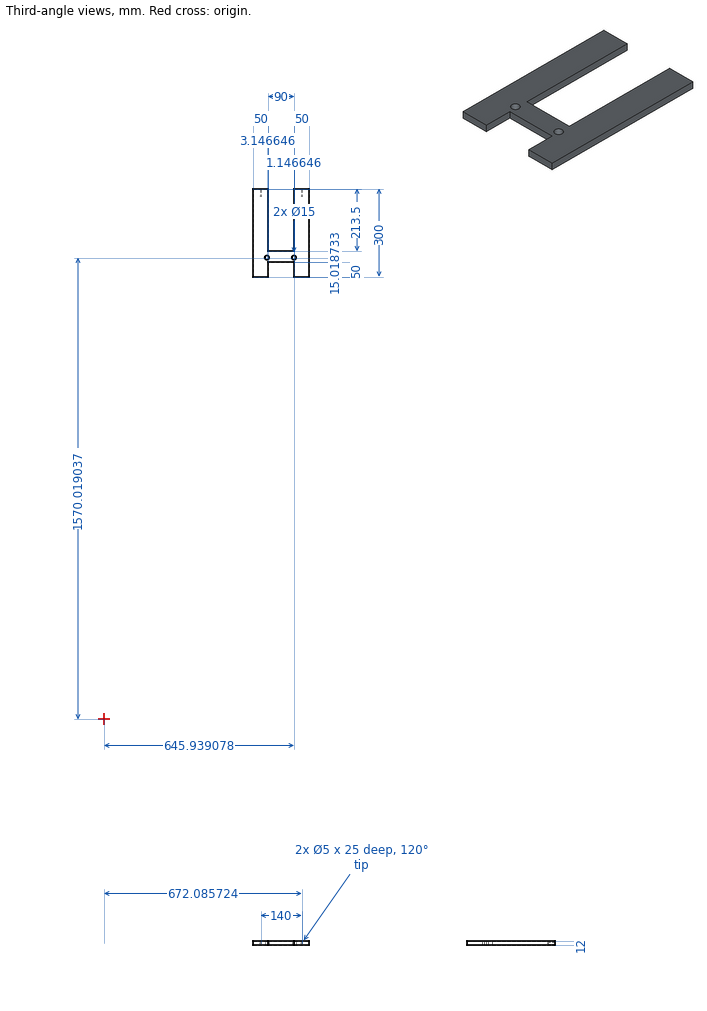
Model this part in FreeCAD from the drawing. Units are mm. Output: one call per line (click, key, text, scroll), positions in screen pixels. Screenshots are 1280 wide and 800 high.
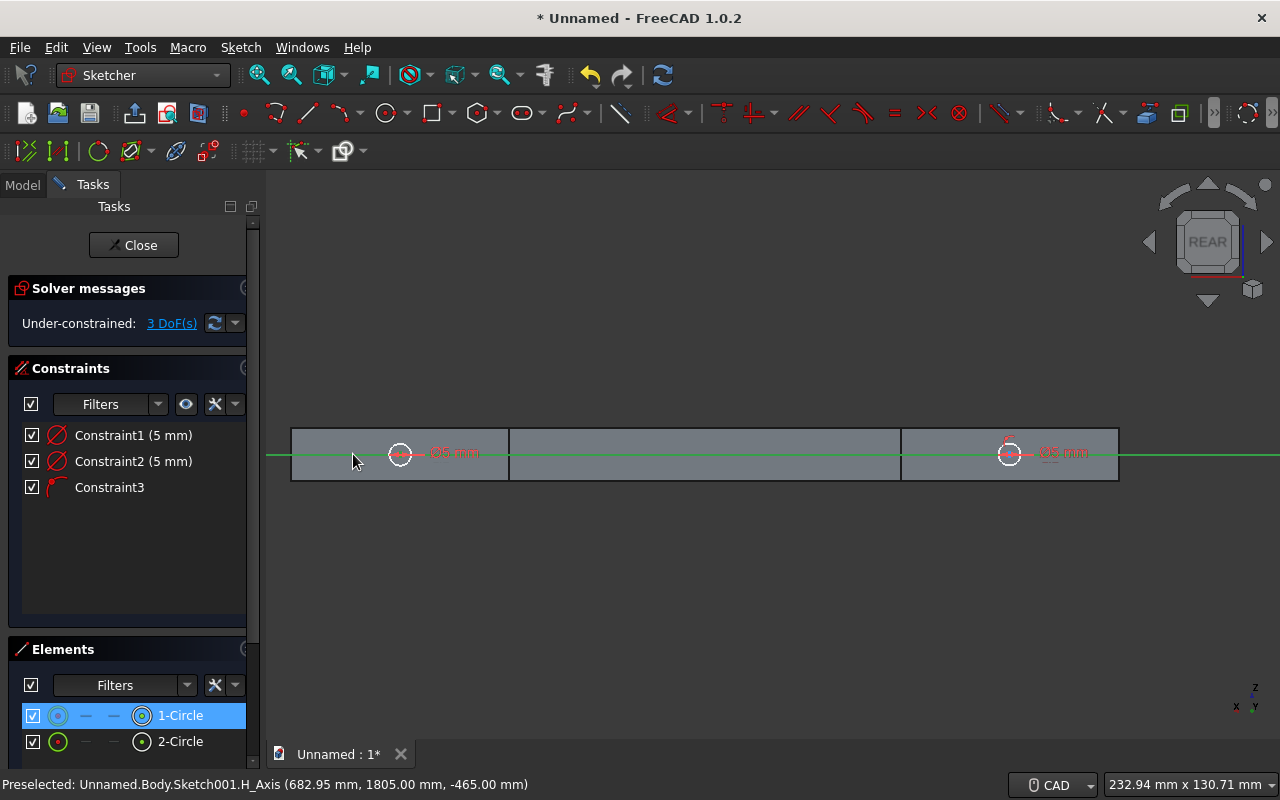
click(722, 114)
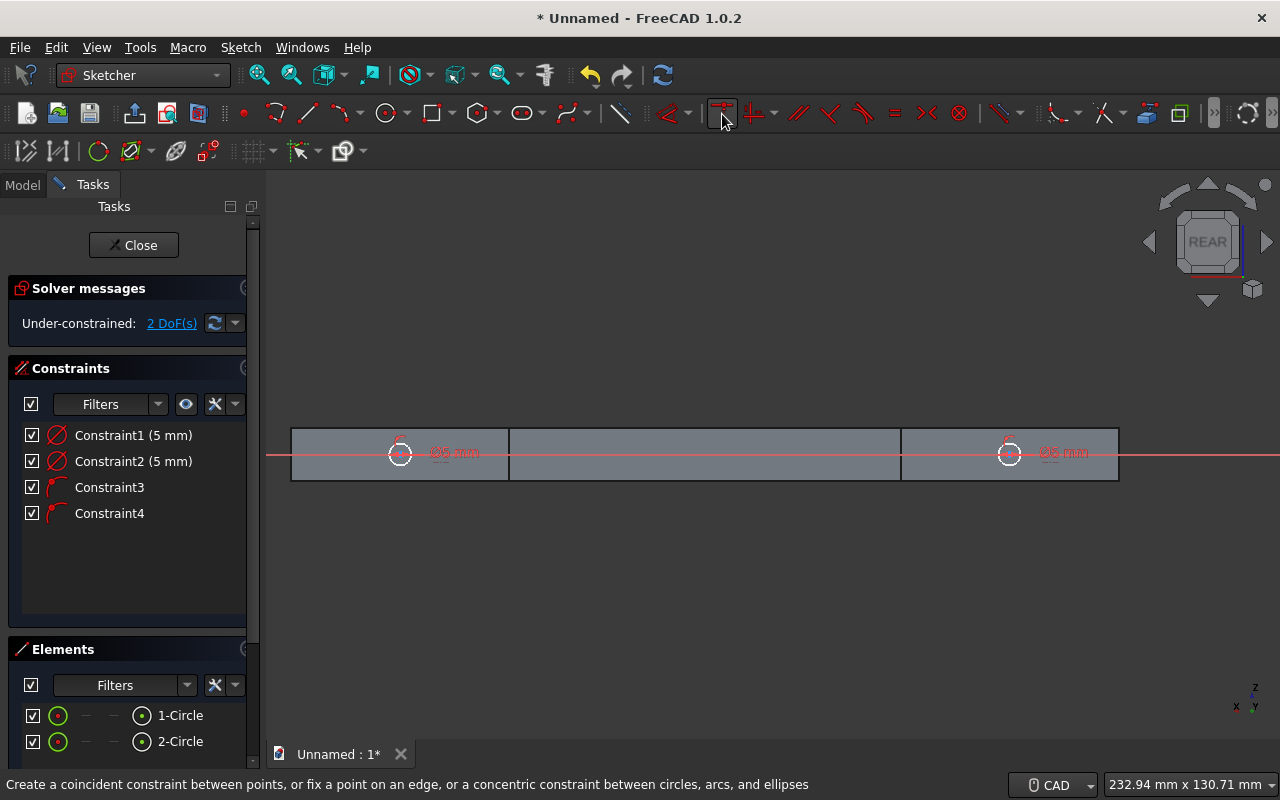
key(d)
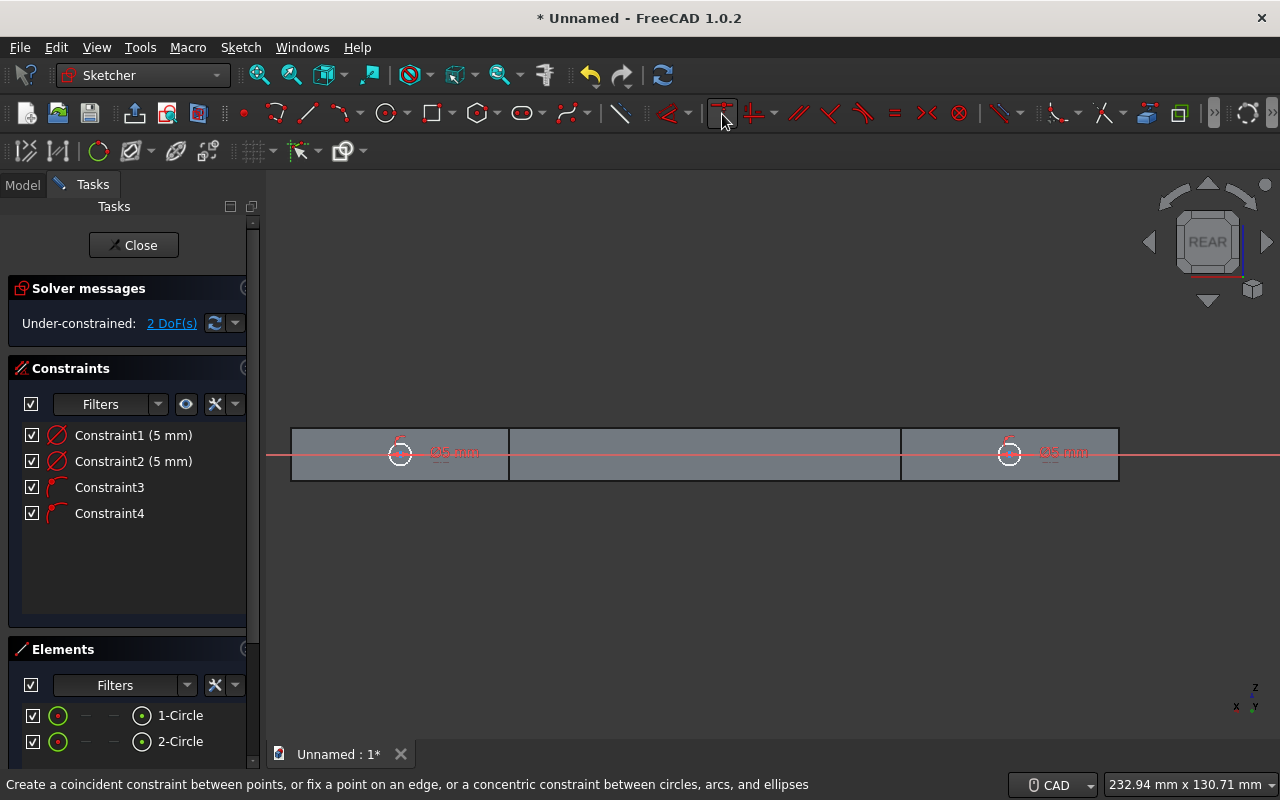
click(400, 454)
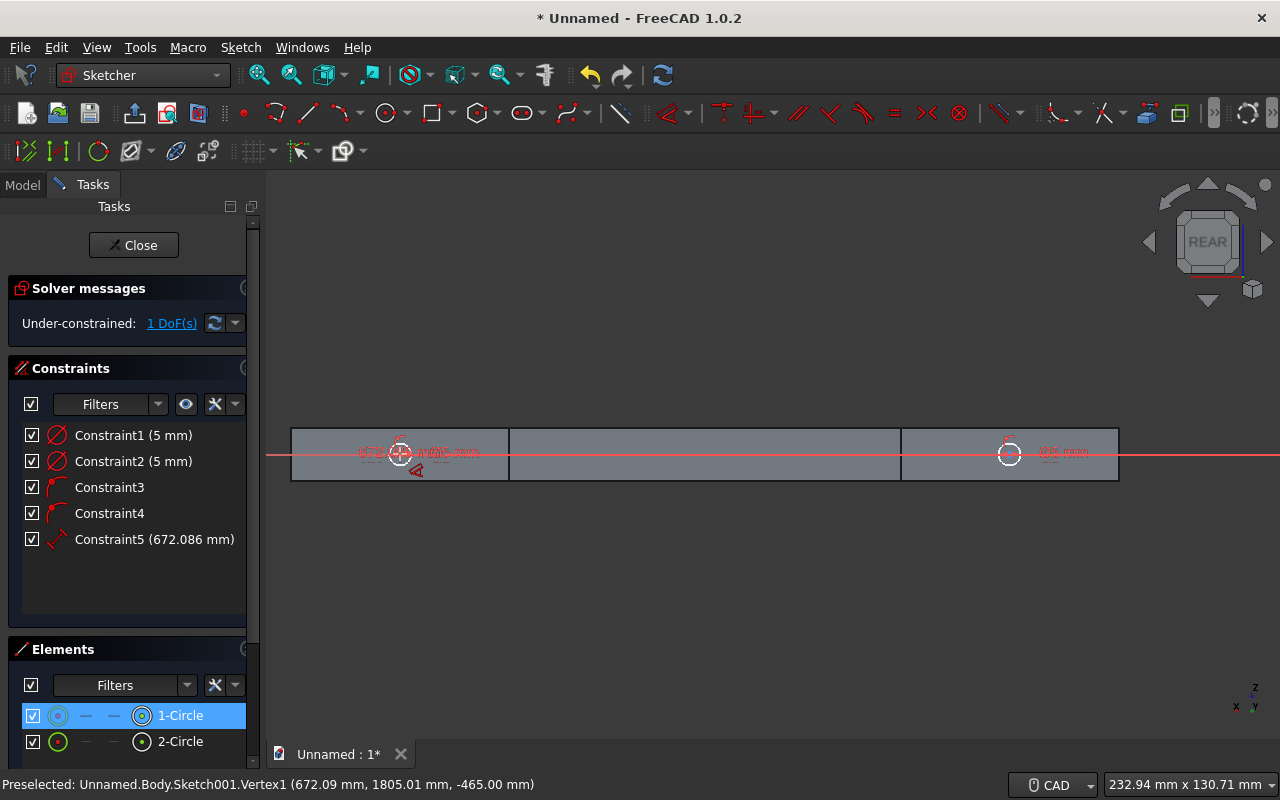
click(1010, 454)
click(705, 488)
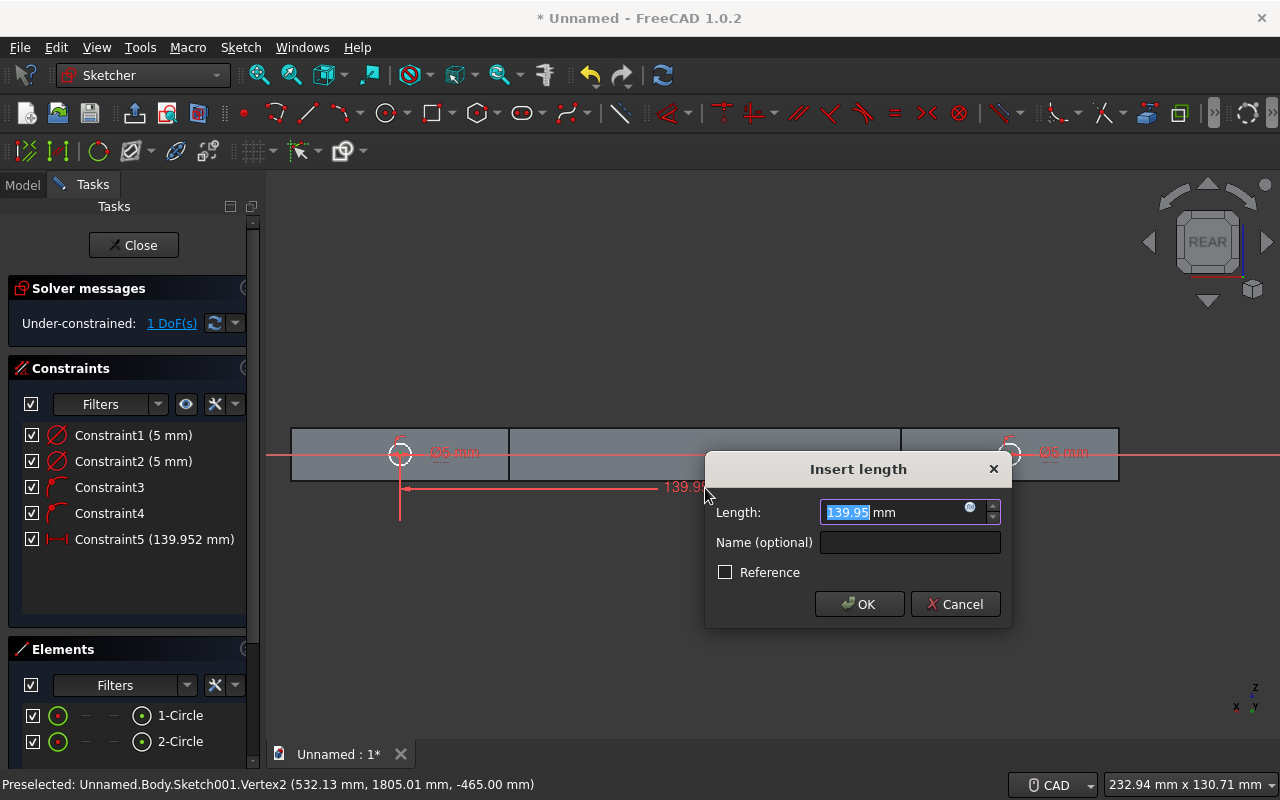
text(140)
key(Return)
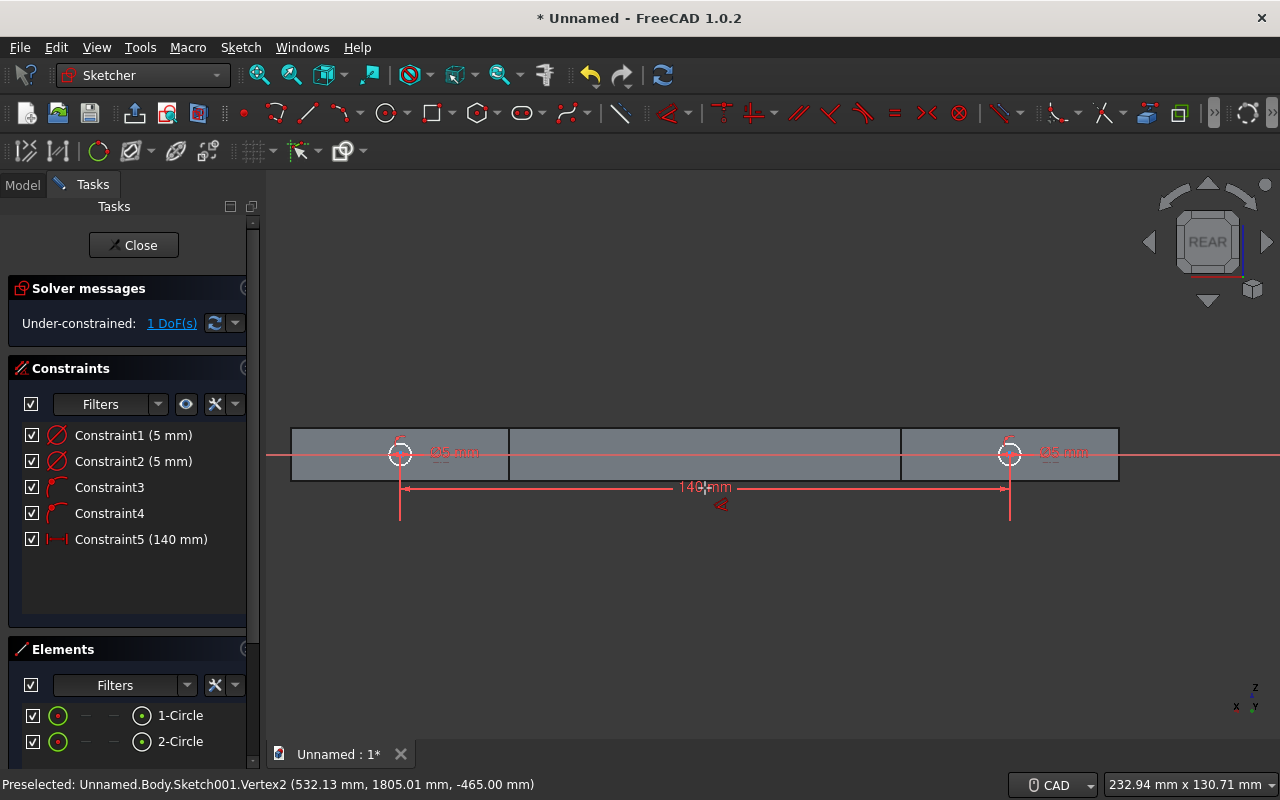
click(400, 454)
click(593, 488)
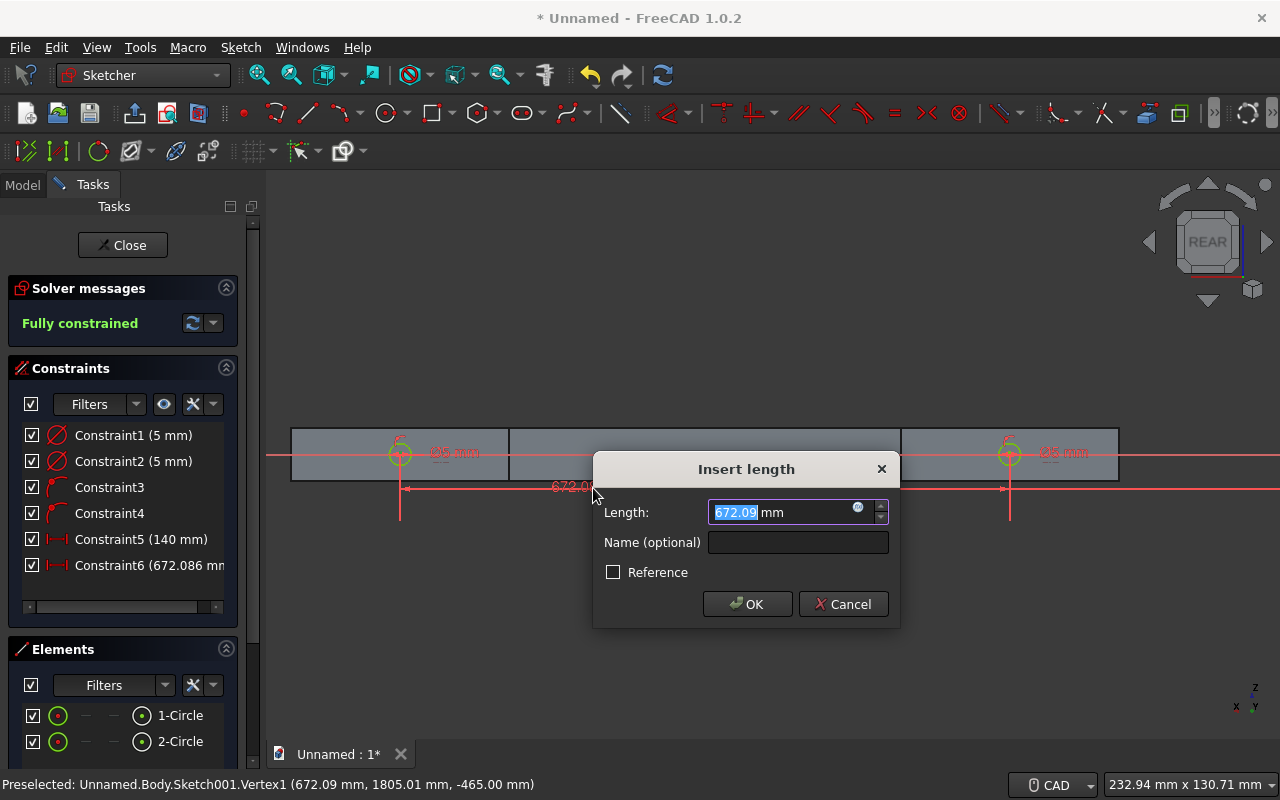
text(672.085724)
key(Return)
key(Escape)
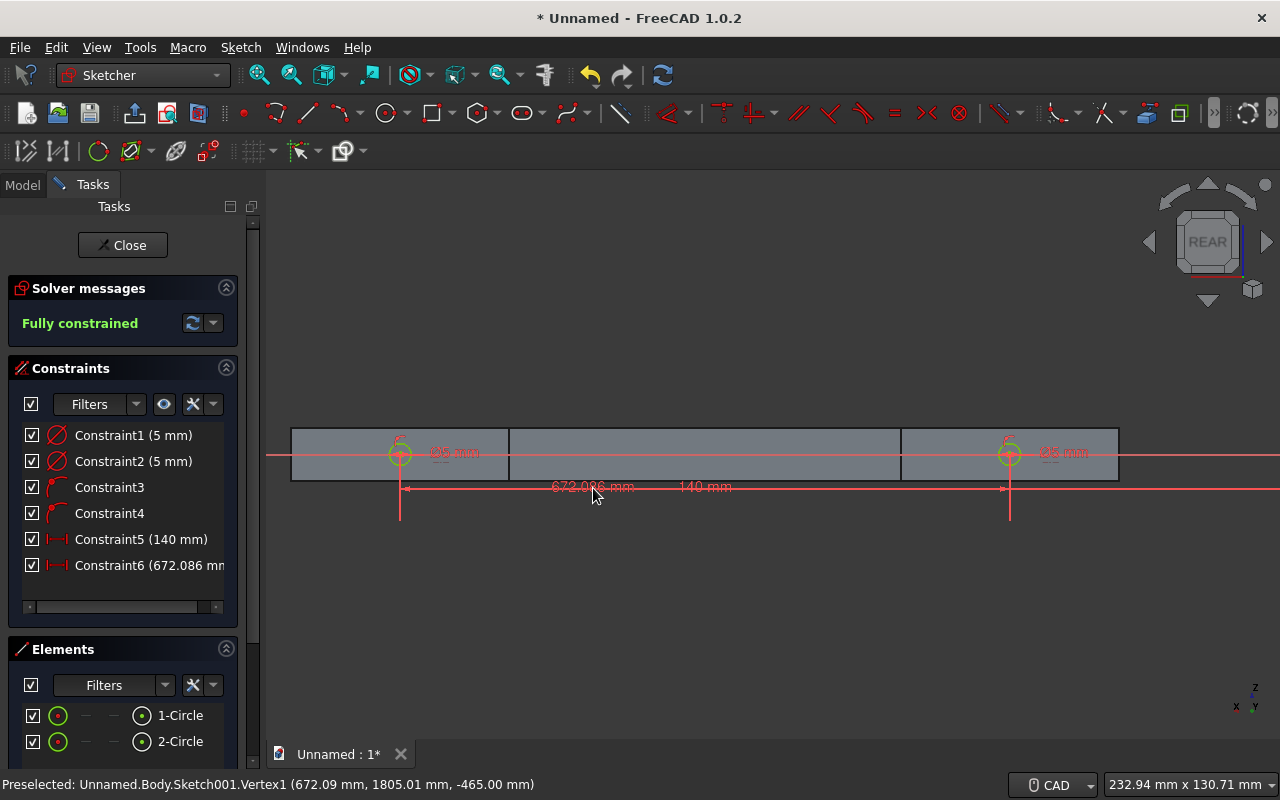
click(123, 245)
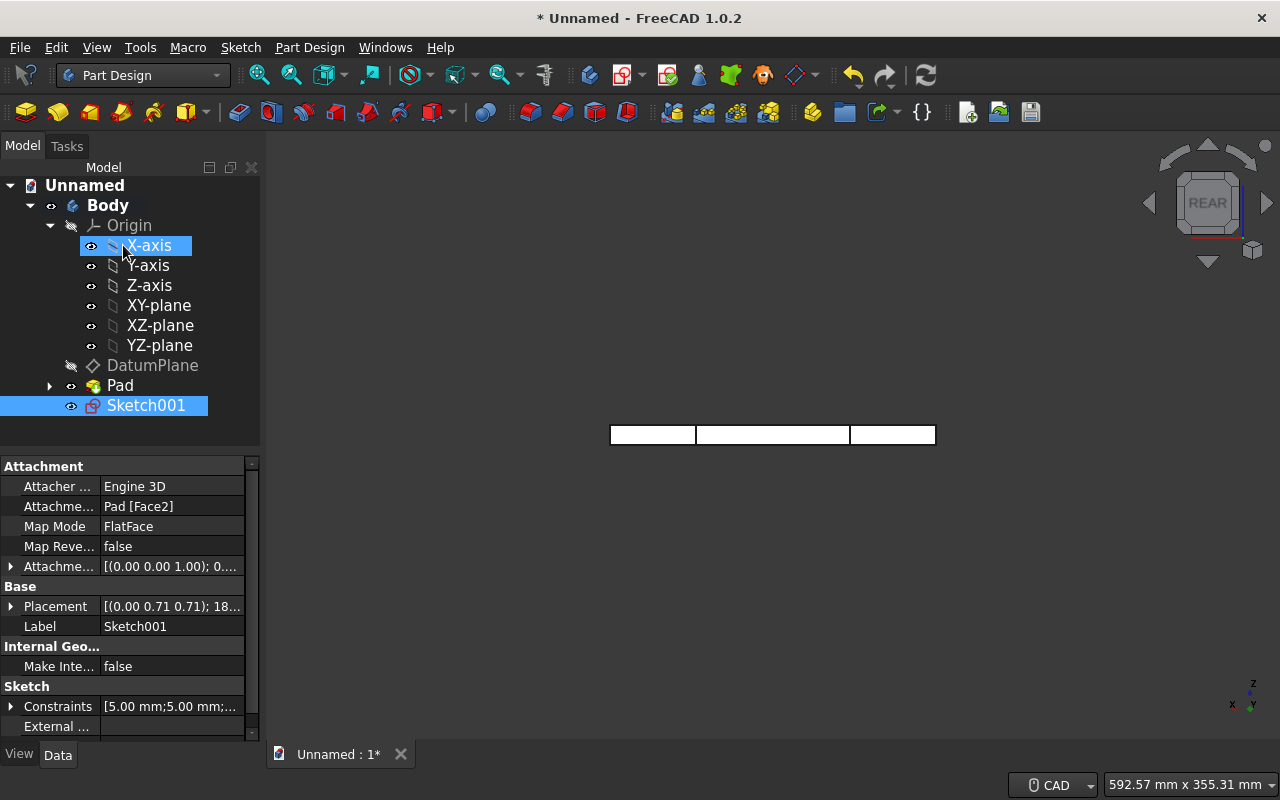
click(272, 112)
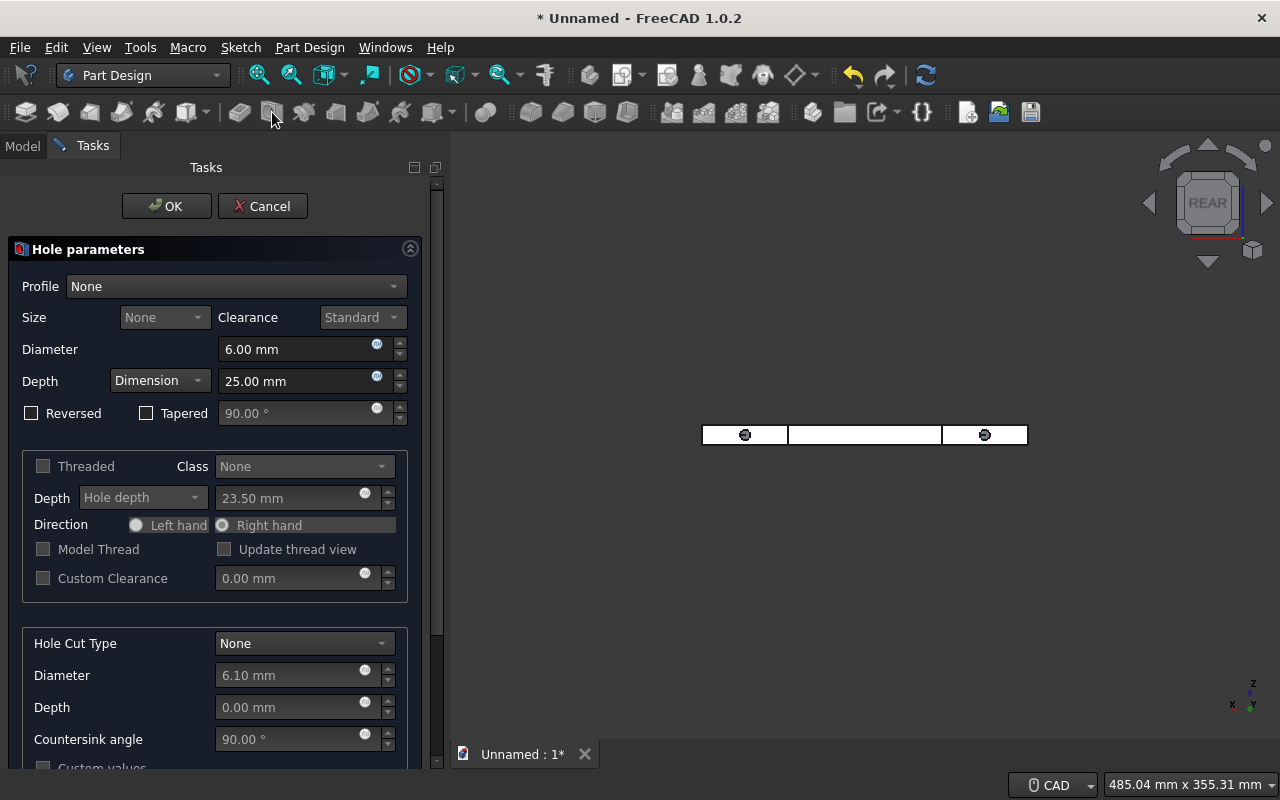
triple_click(305, 349)